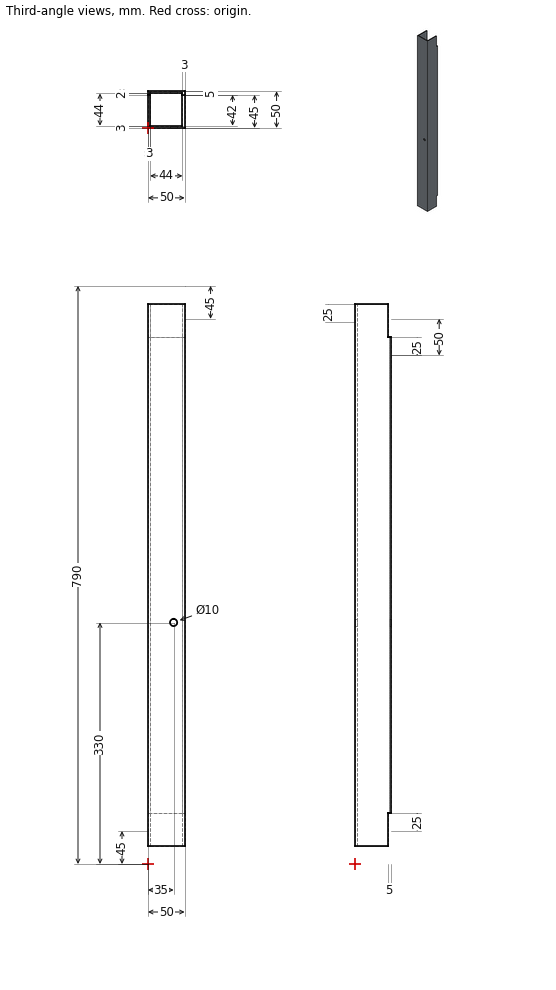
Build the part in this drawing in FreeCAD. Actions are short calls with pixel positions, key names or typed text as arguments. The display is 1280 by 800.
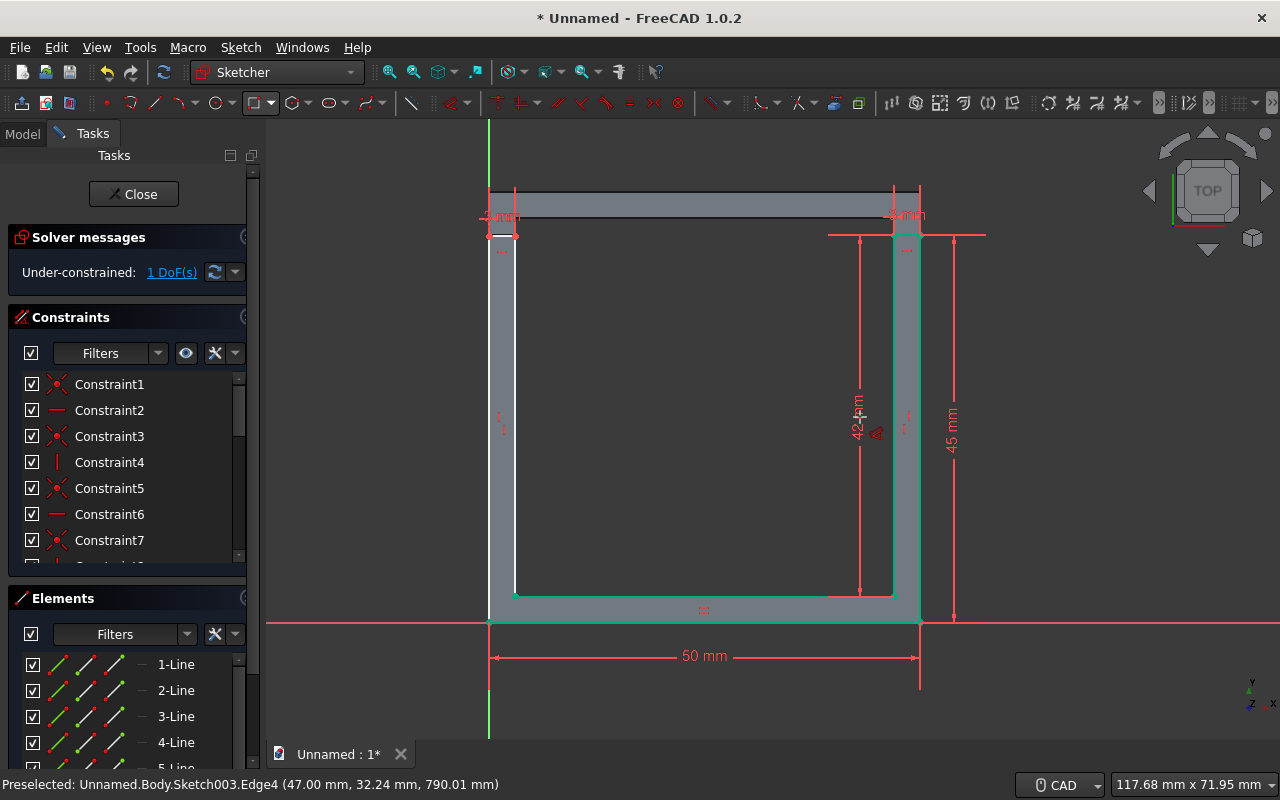
click(515, 489)
click(549, 417)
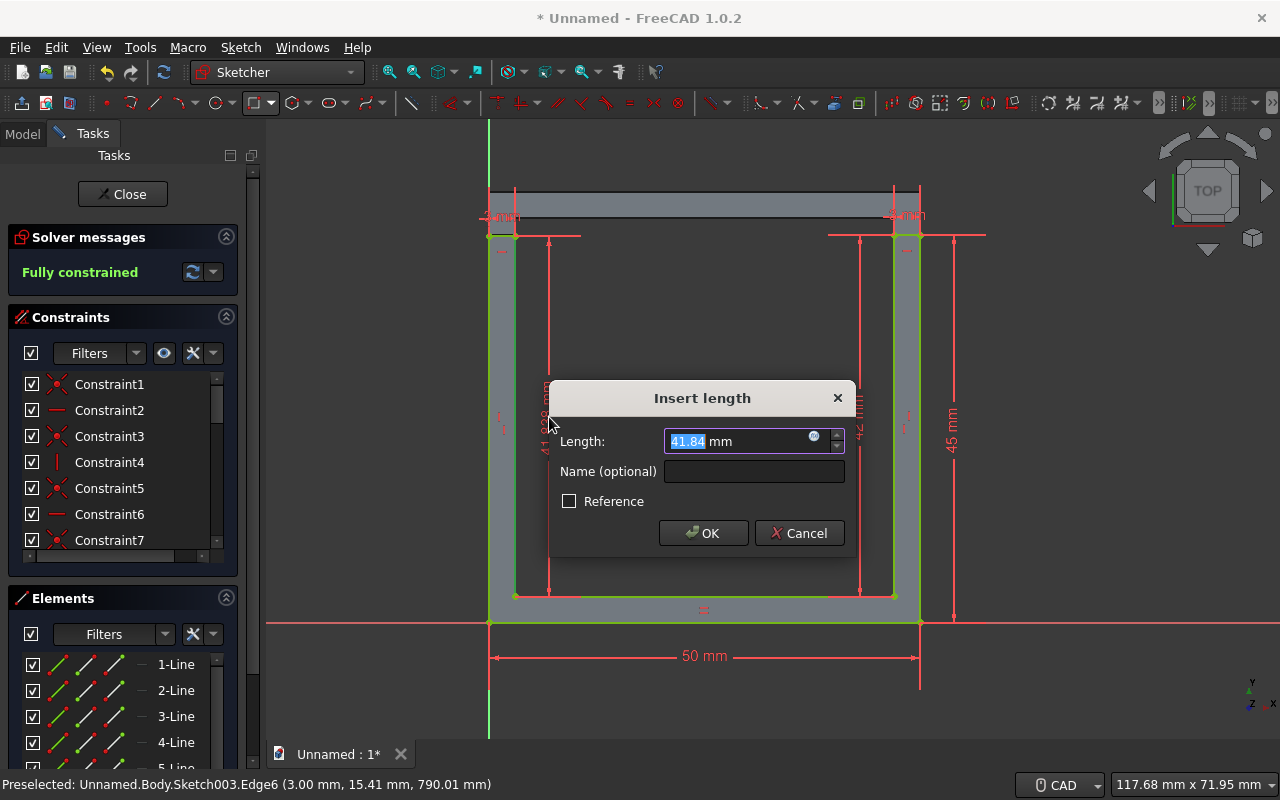
text(42)
key(Return)
key(Escape)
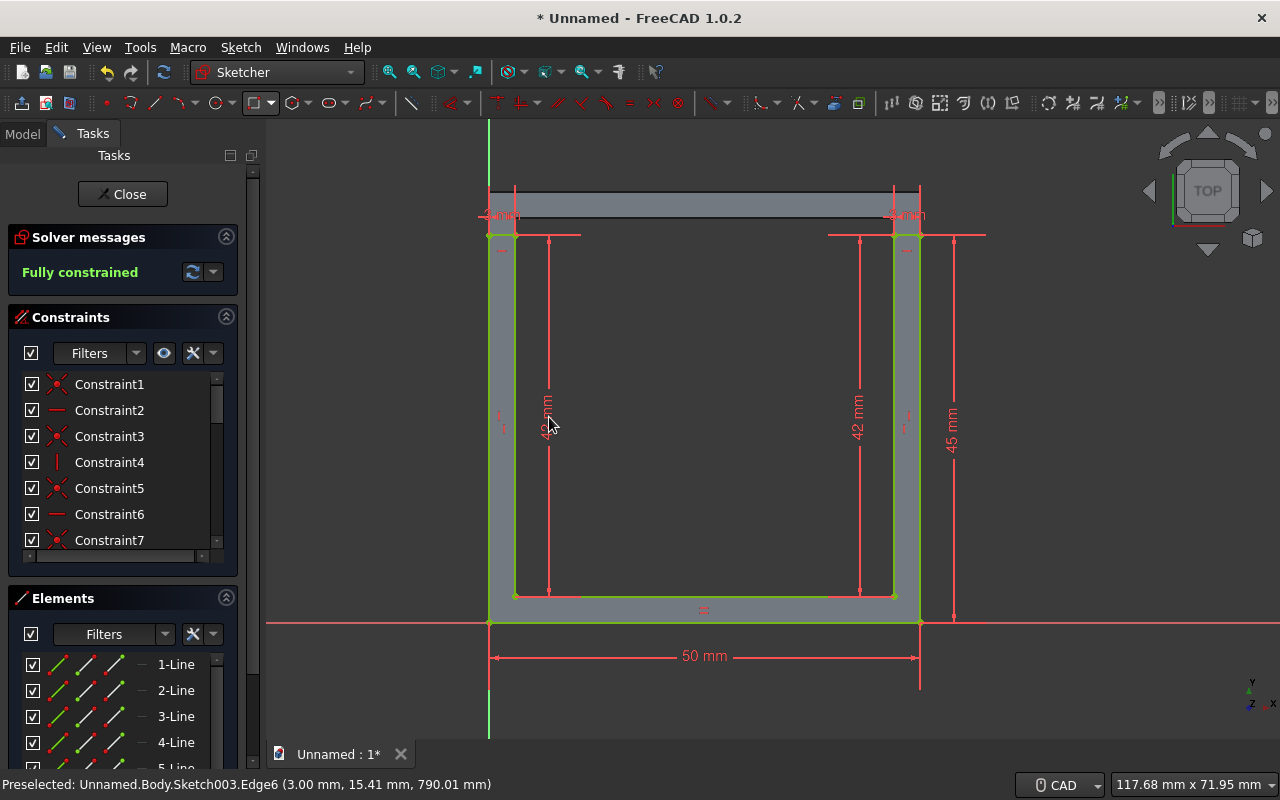
click(123, 194)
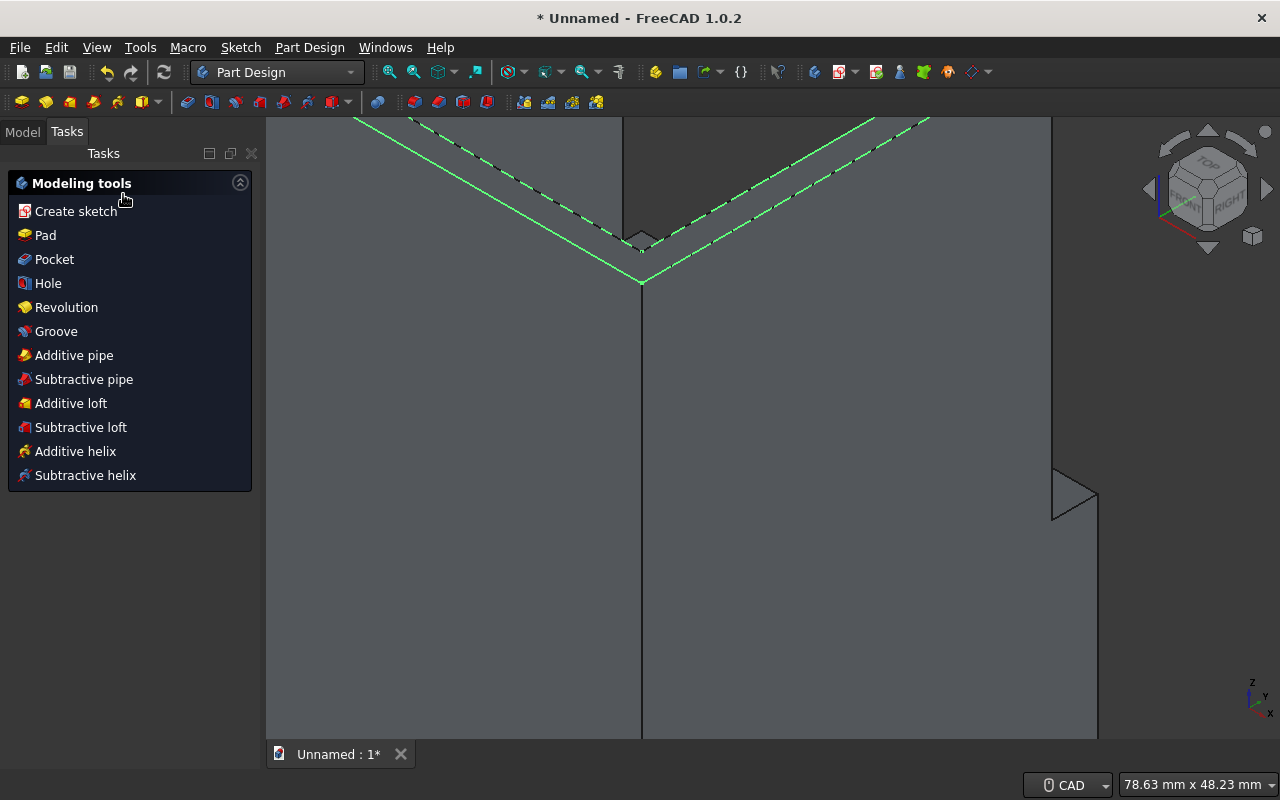
click(188, 102)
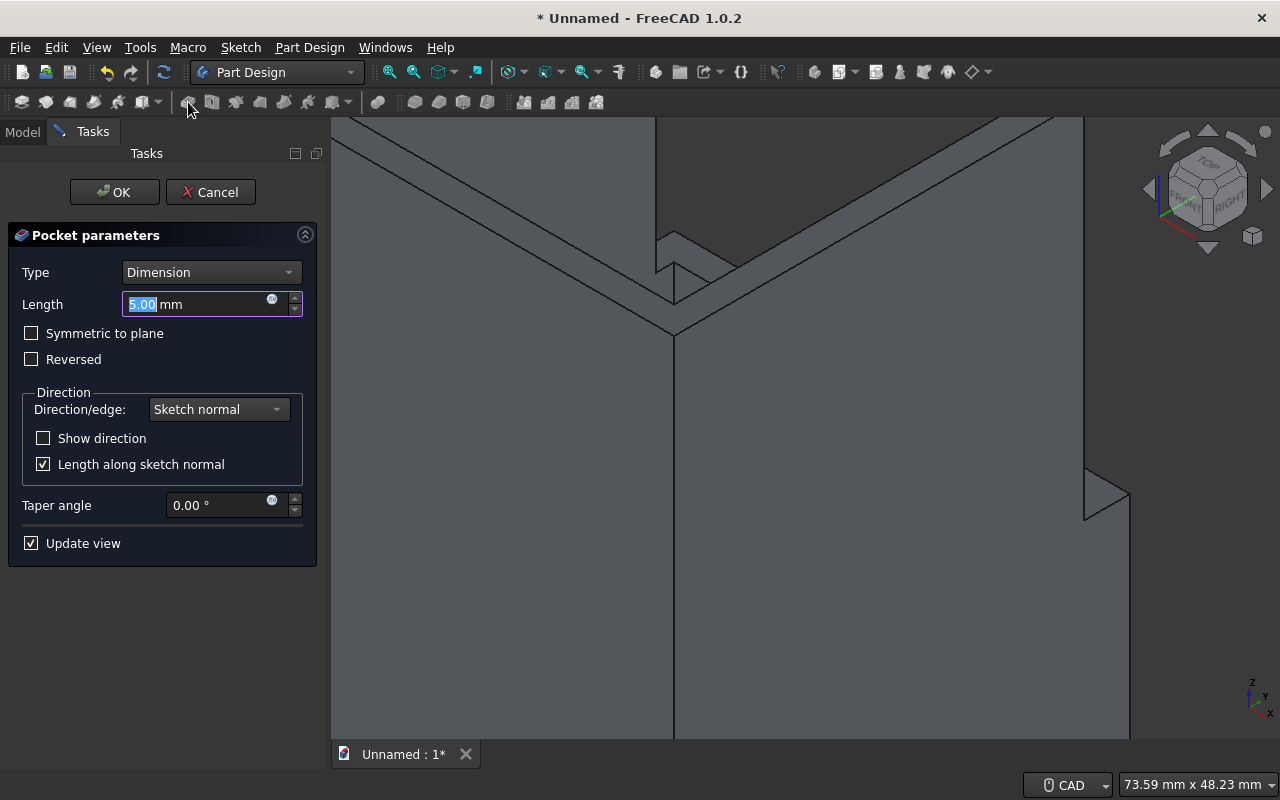
text(50)
key(Tab)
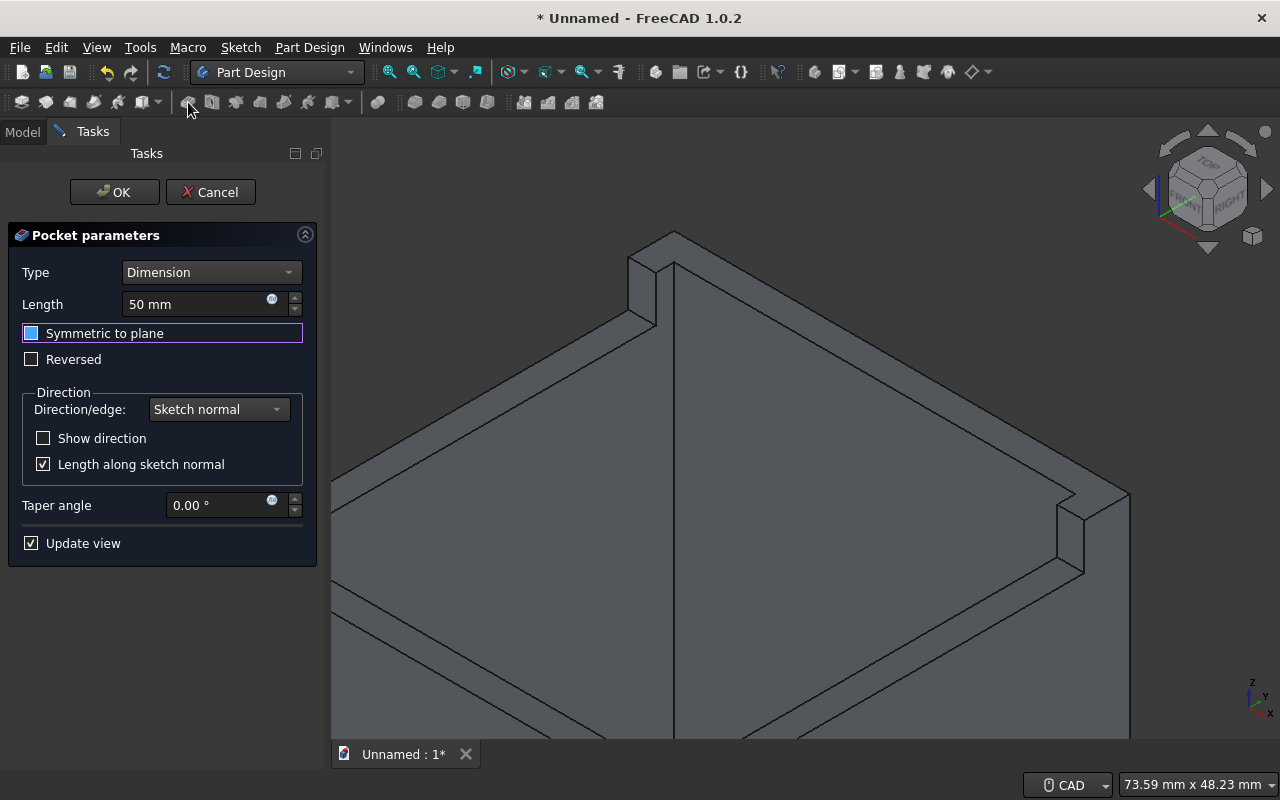
click(115, 192)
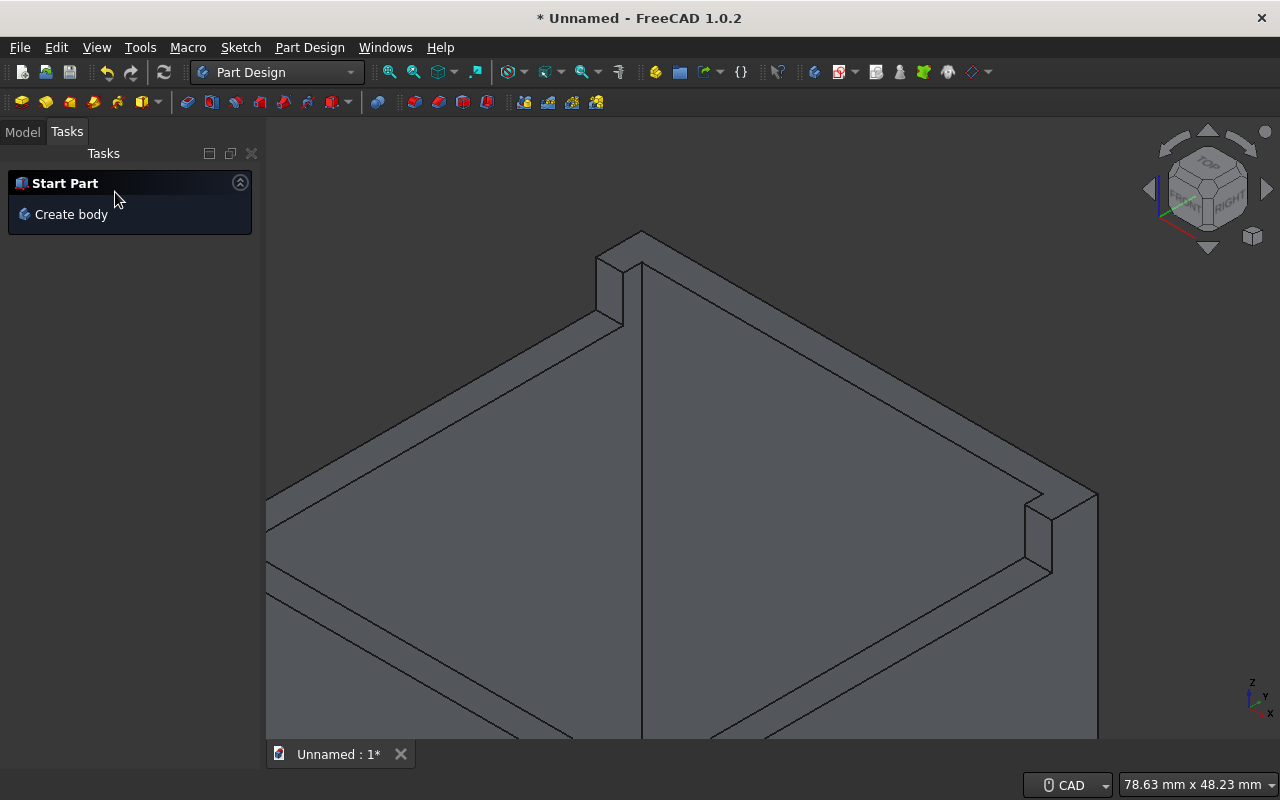
click(390, 72)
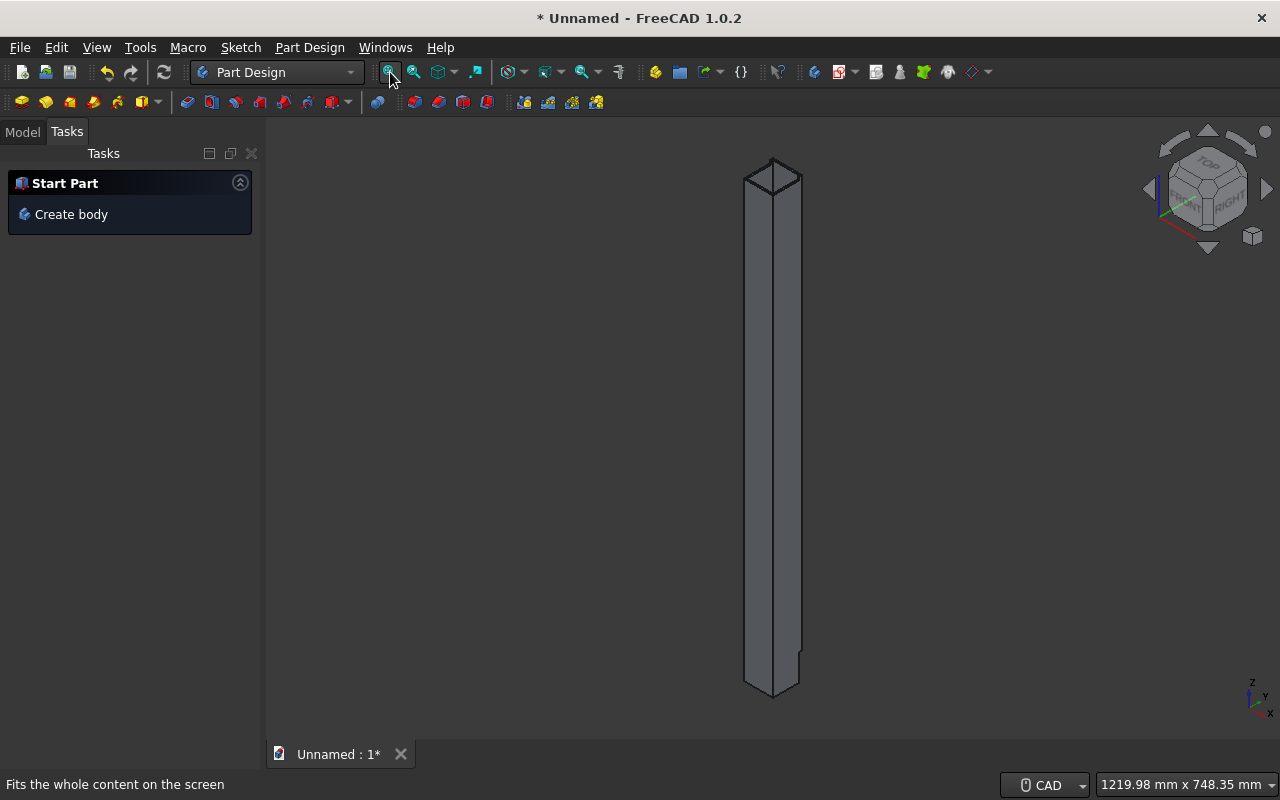
scroll(799, 174, up, 13)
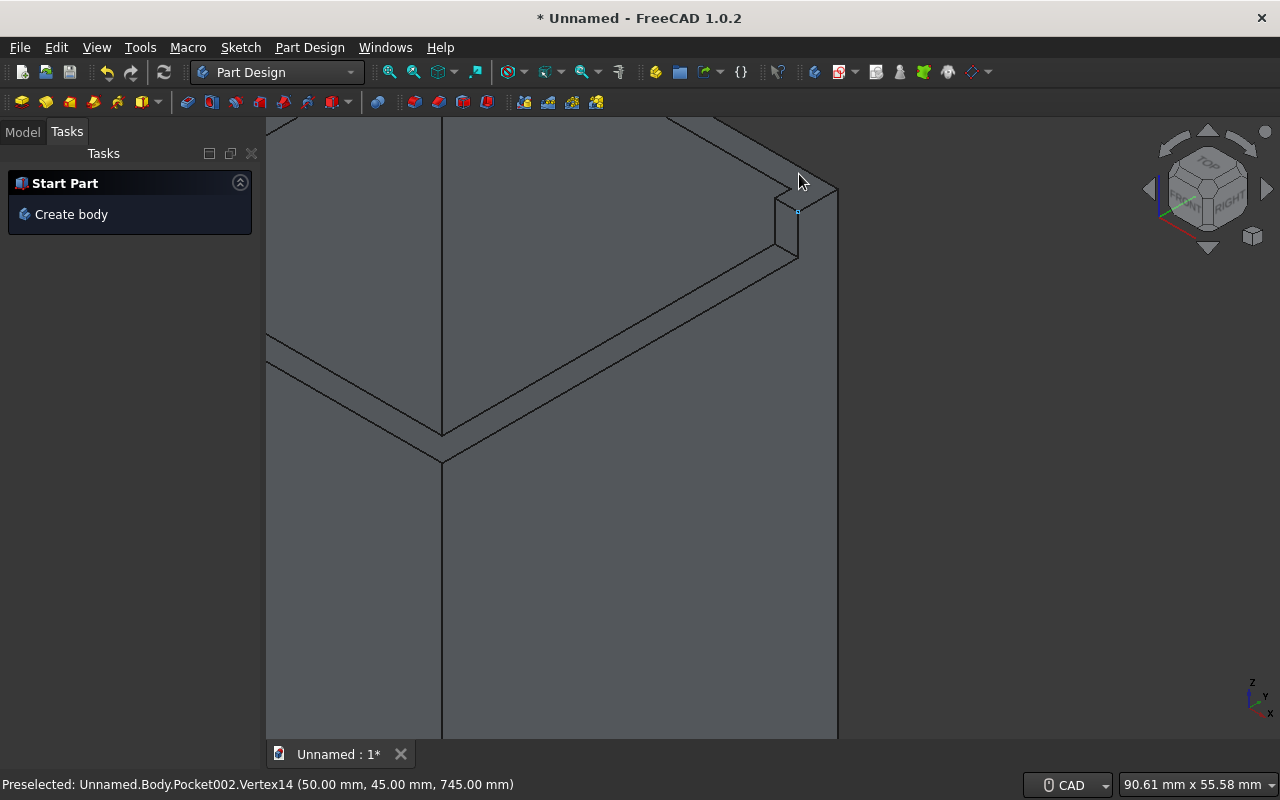
click(796, 180)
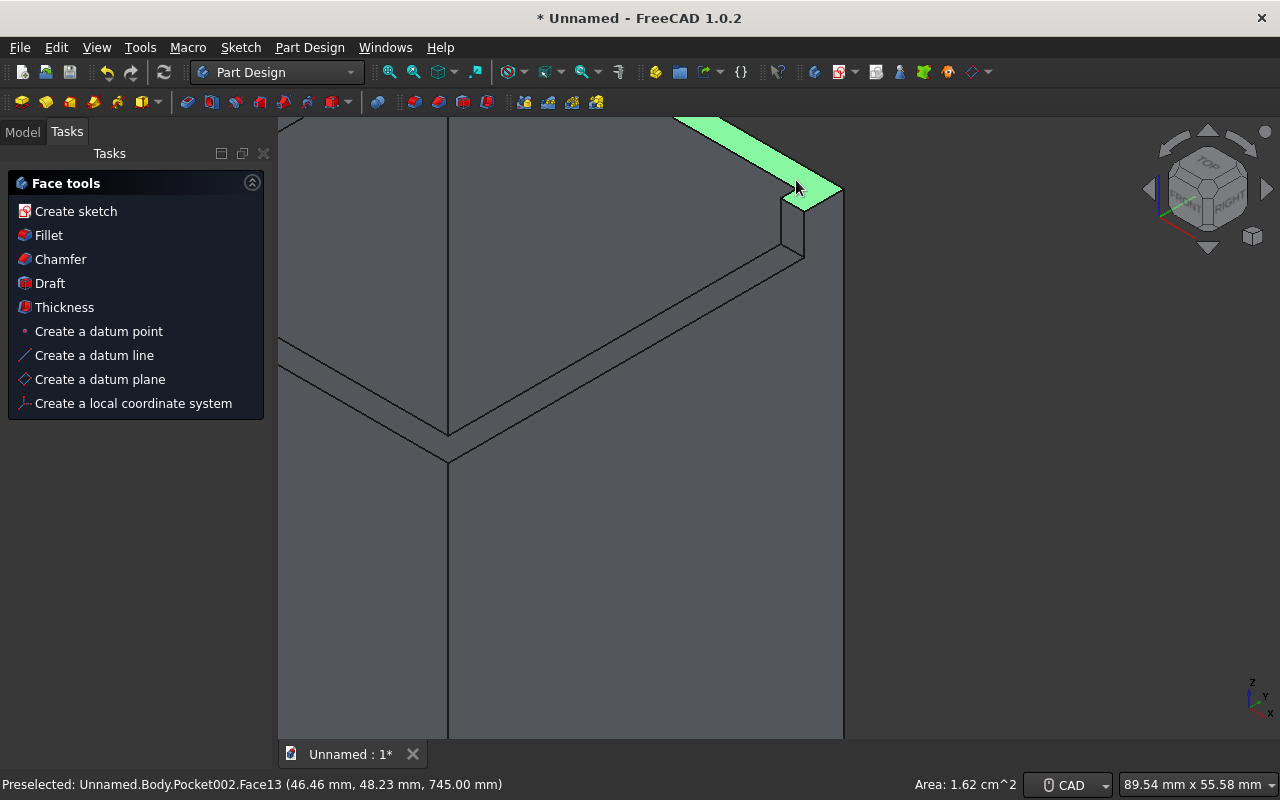
click(840, 72)